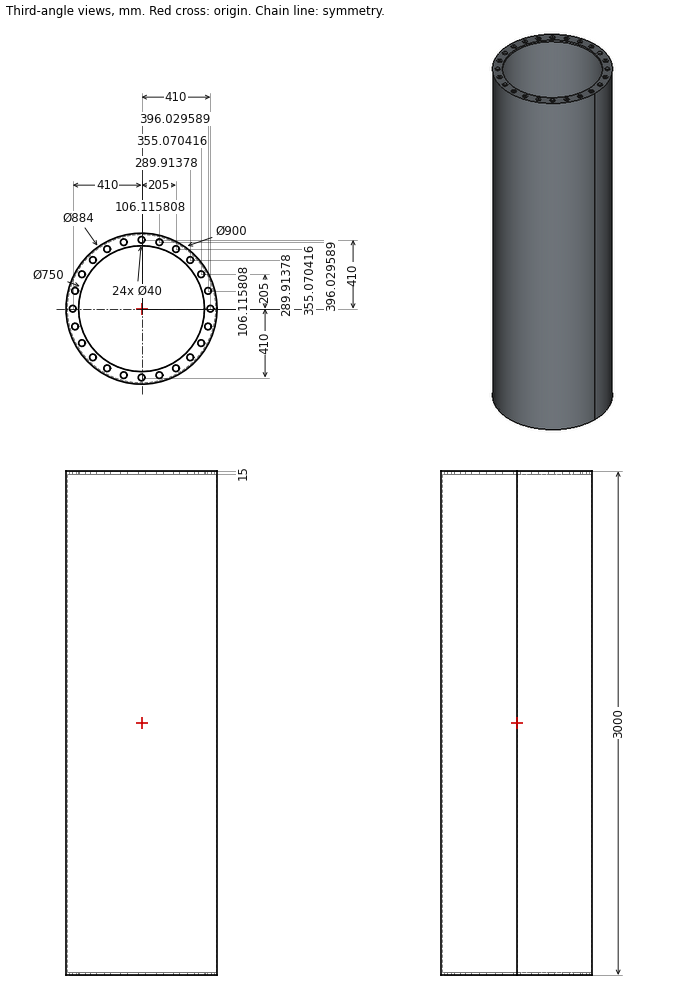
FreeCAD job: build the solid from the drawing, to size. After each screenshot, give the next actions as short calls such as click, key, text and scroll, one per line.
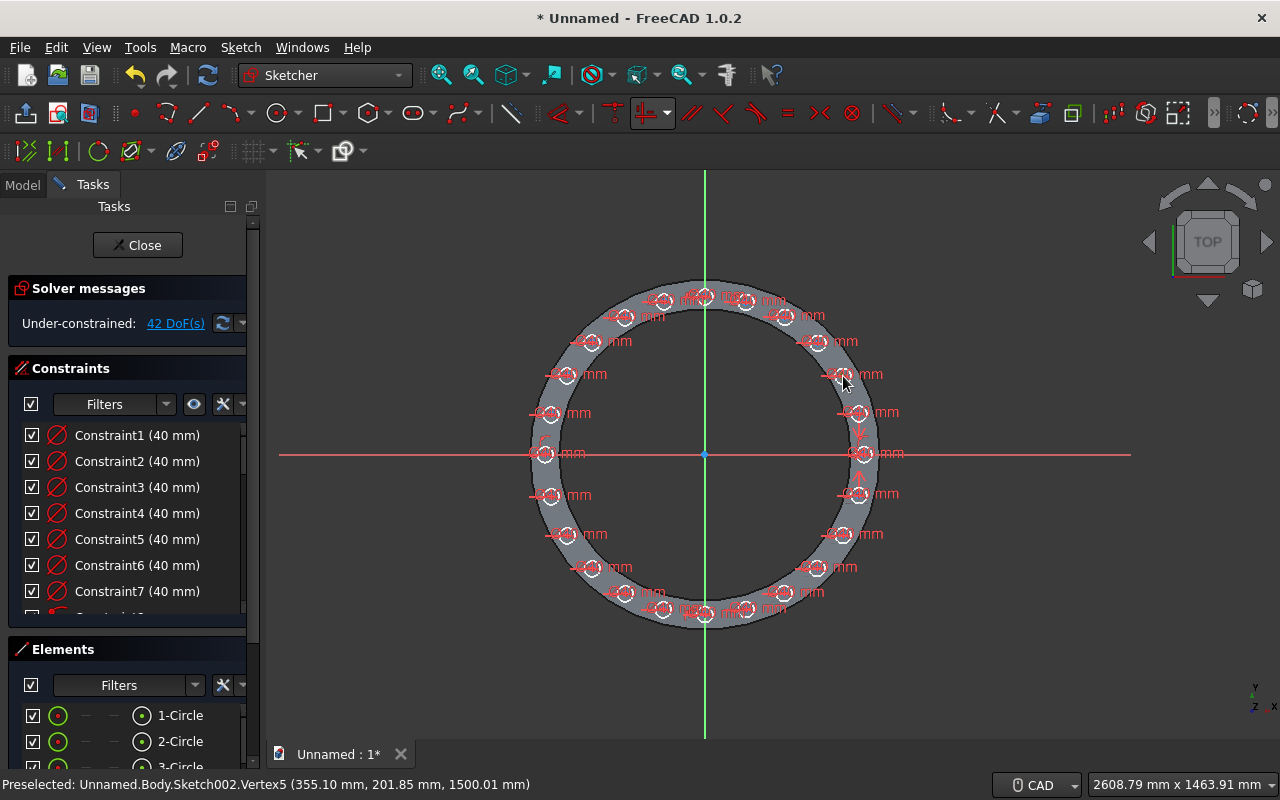
click(843, 536)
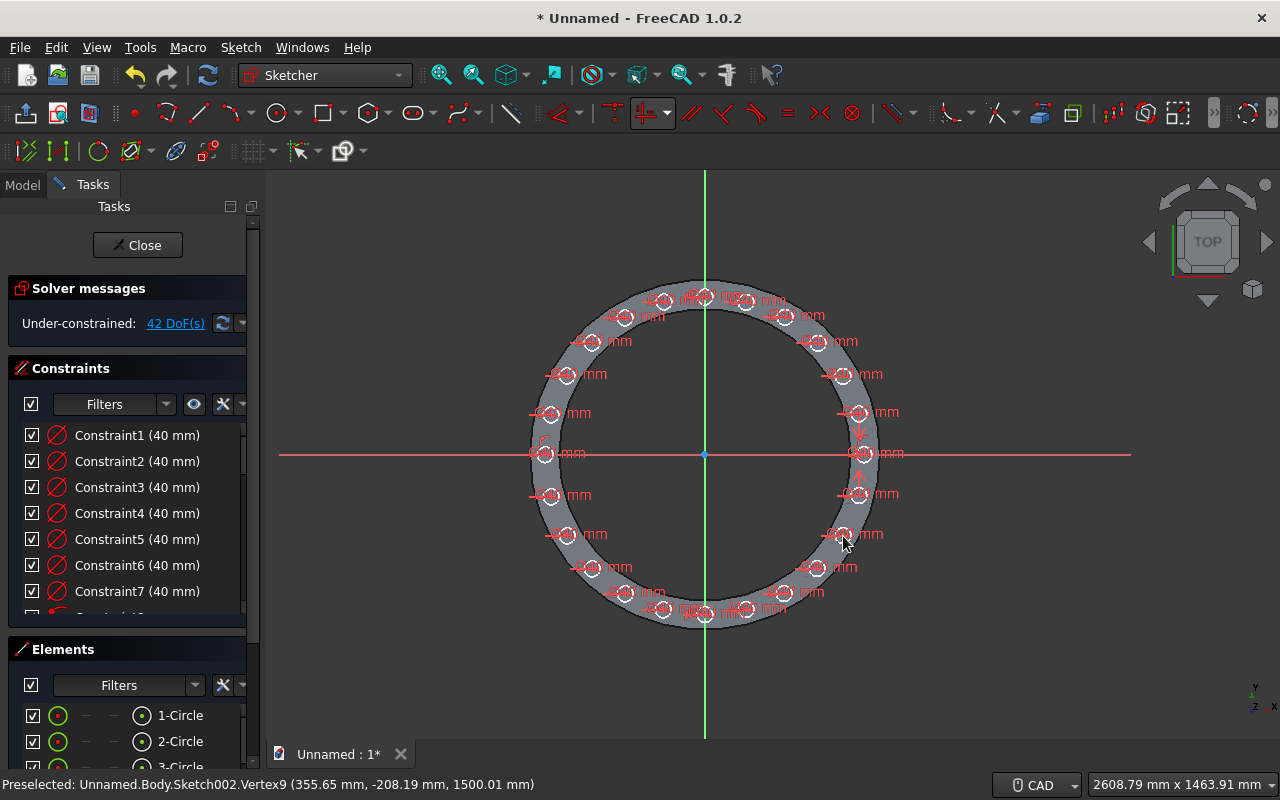
click(353, 455)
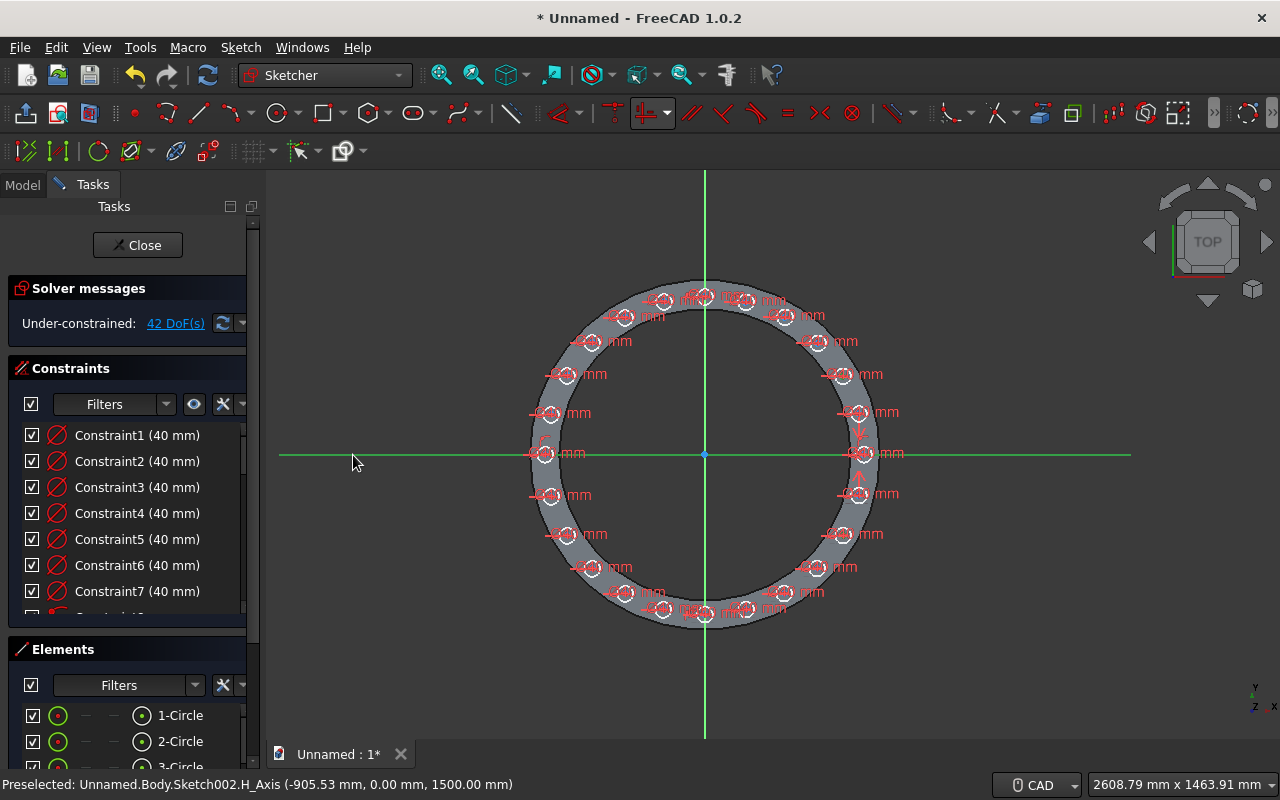
click(820, 114)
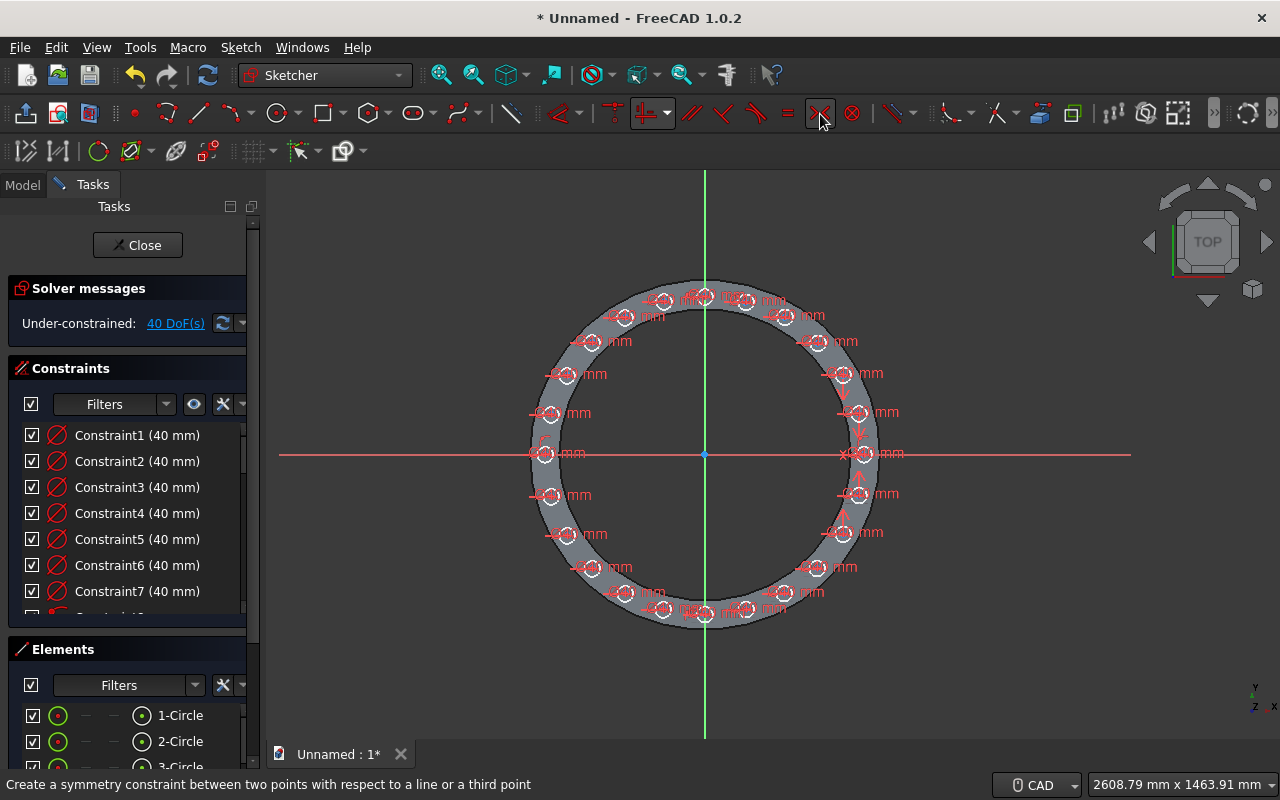
click(818, 343)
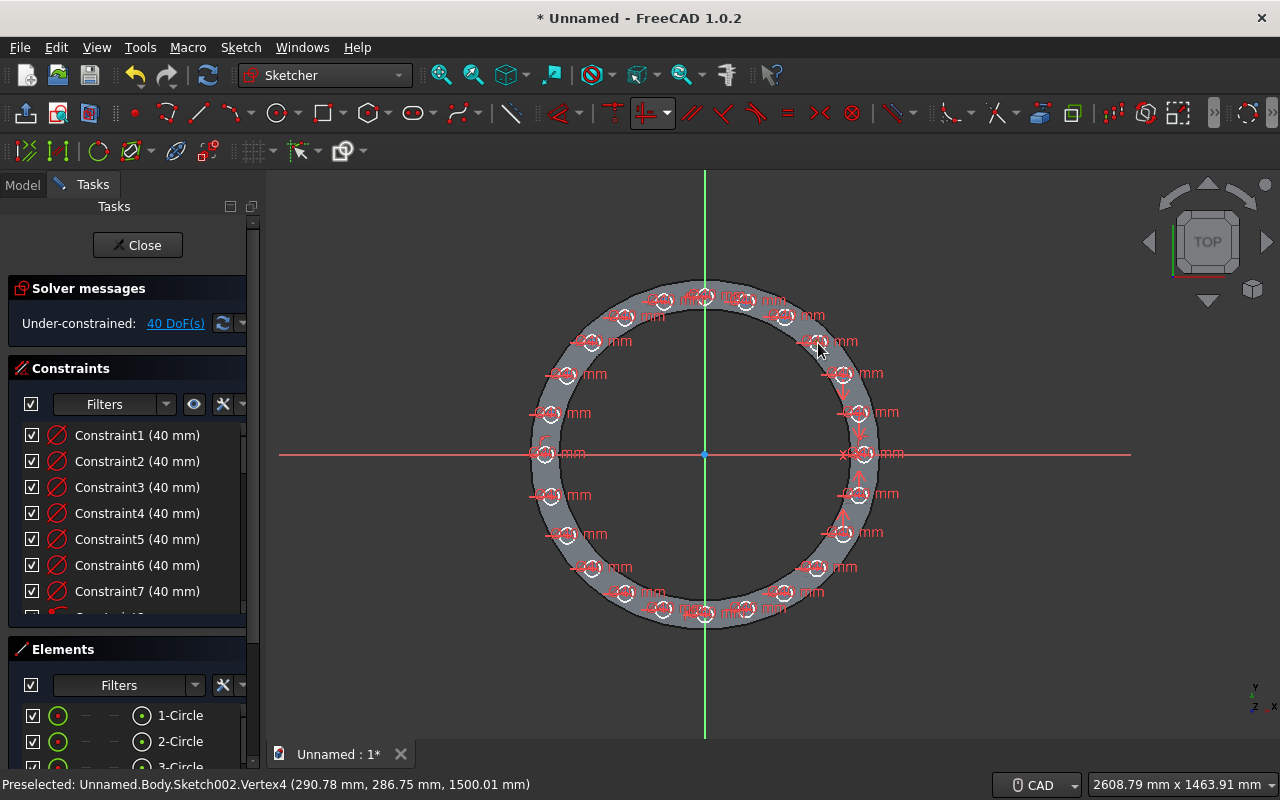
click(817, 569)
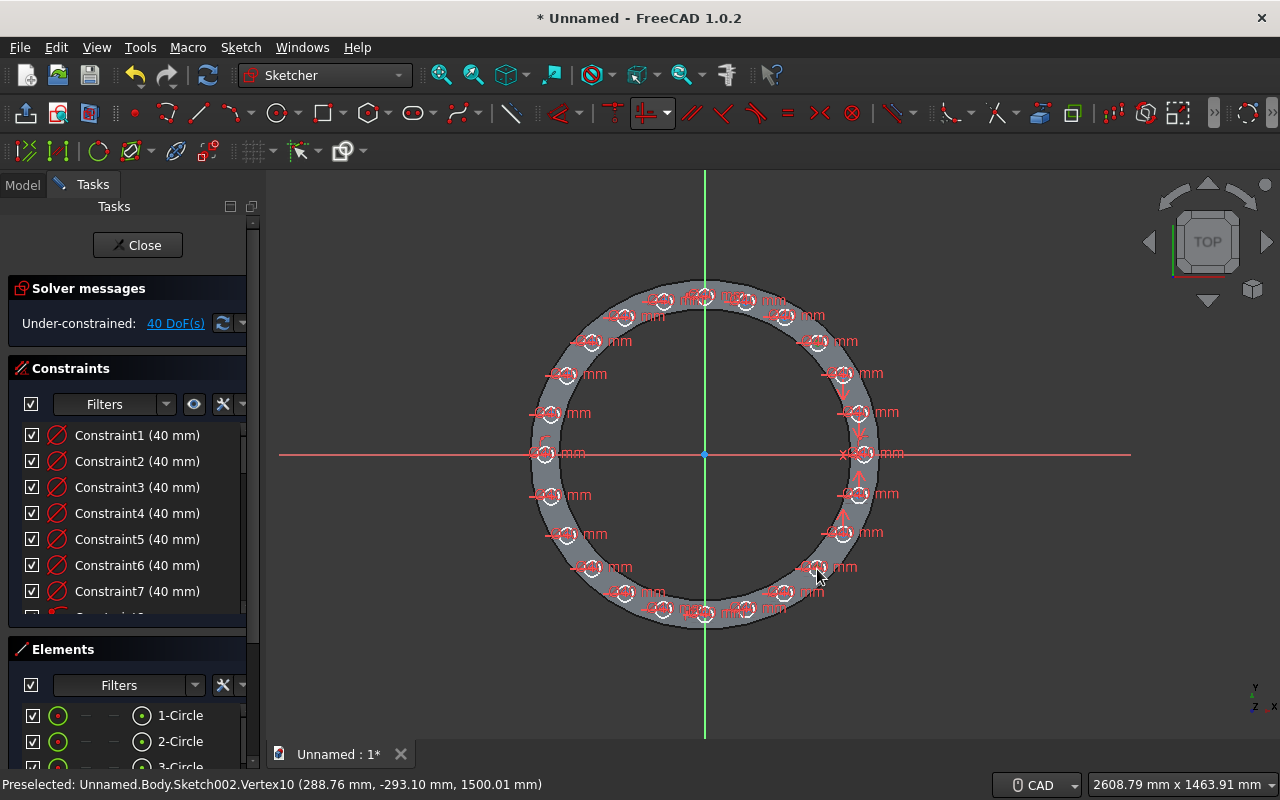
click(353, 455)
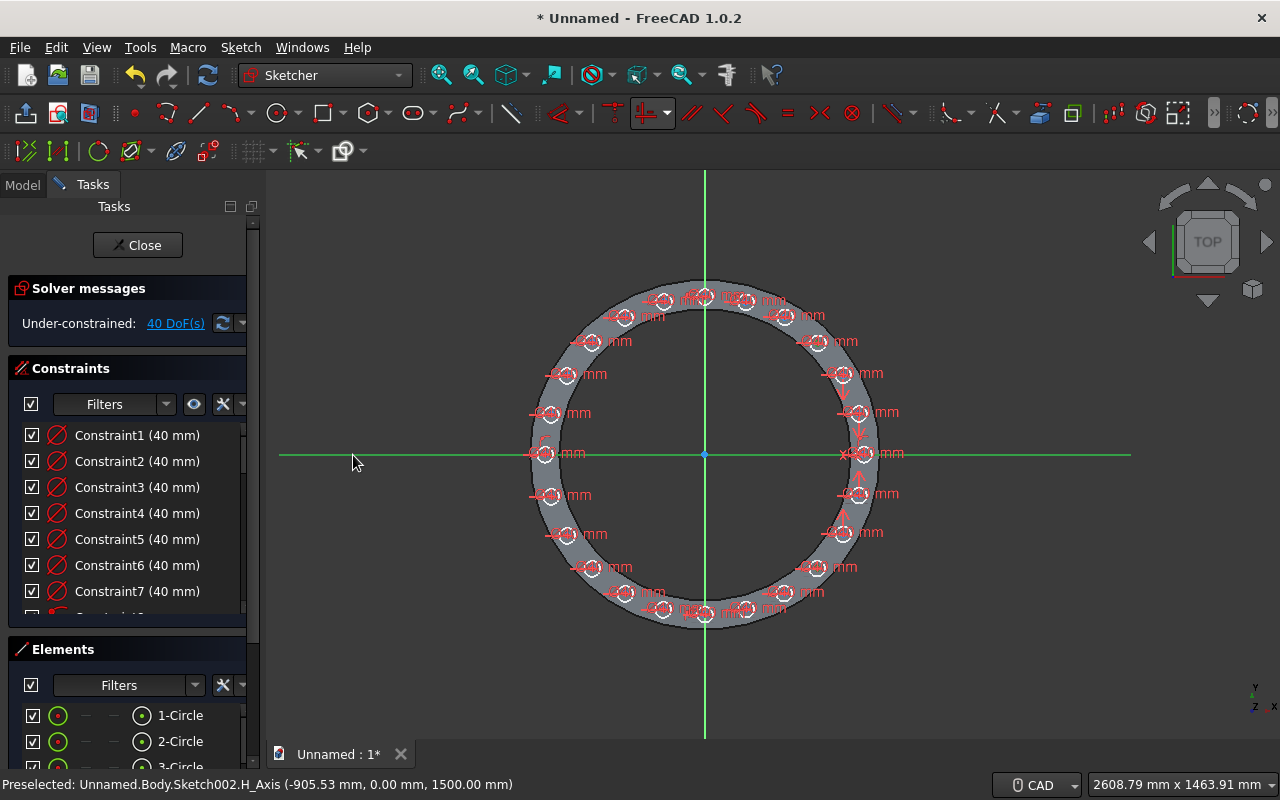
click(820, 114)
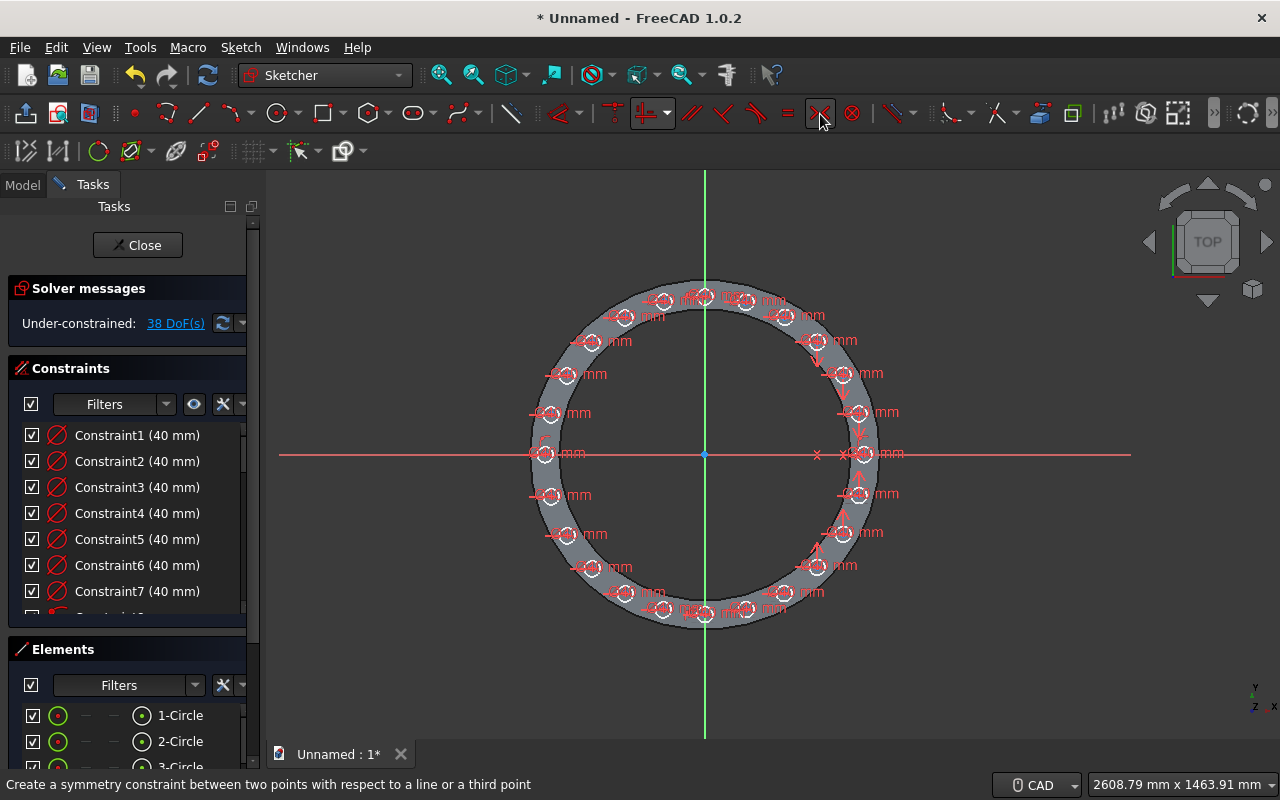
click(785, 317)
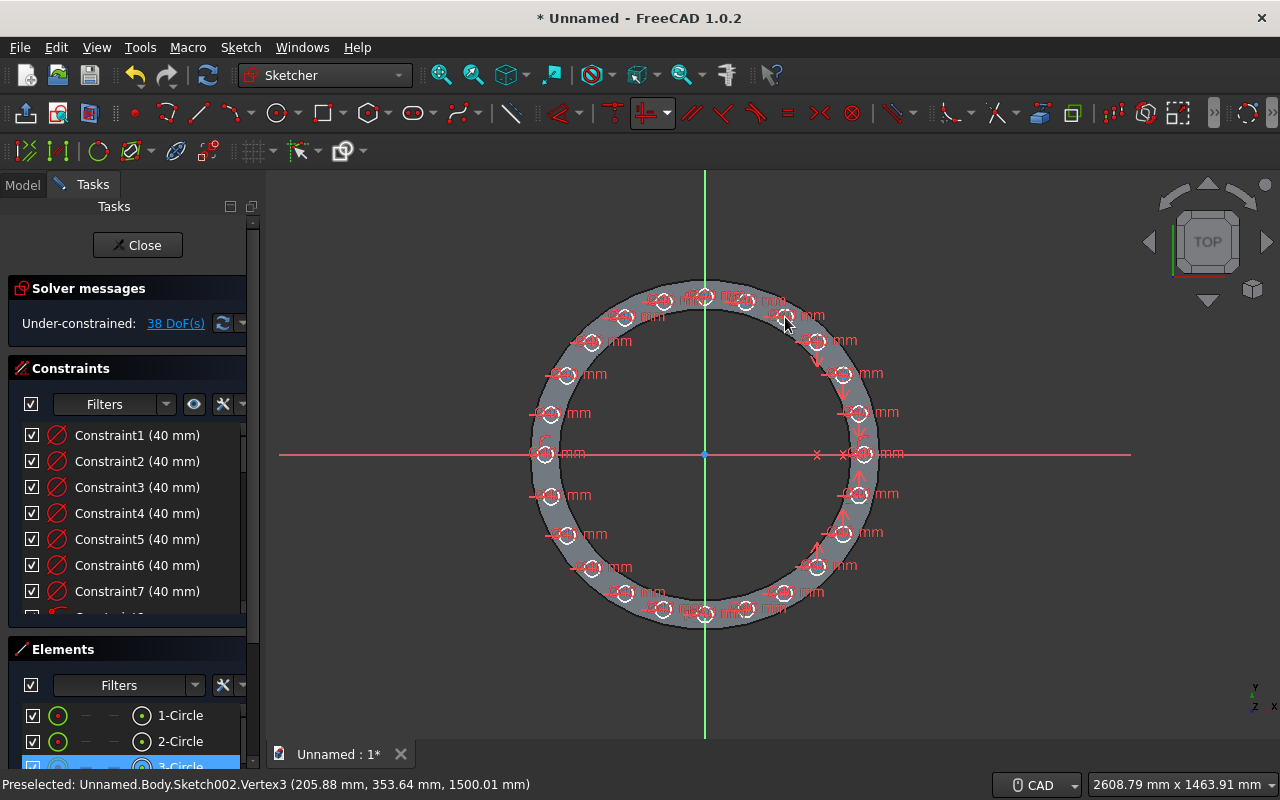
click(784, 594)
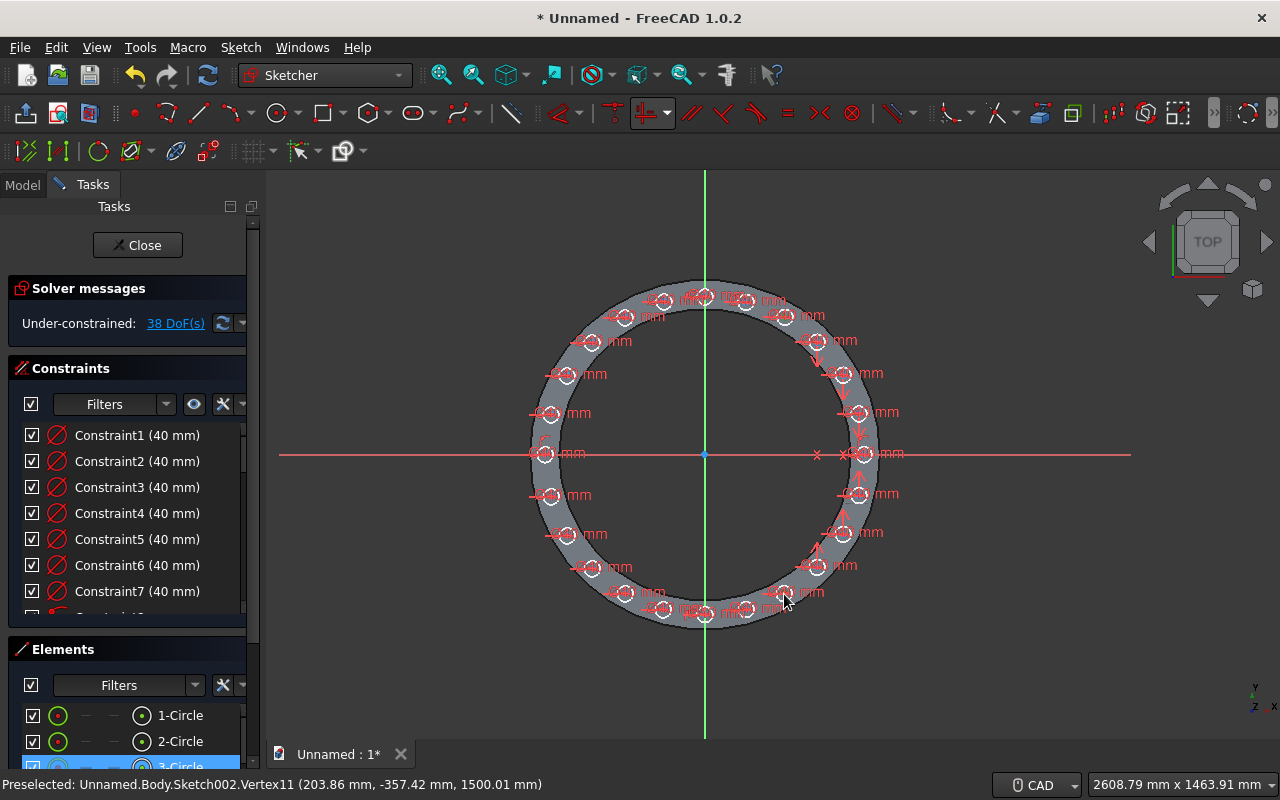
click(353, 455)